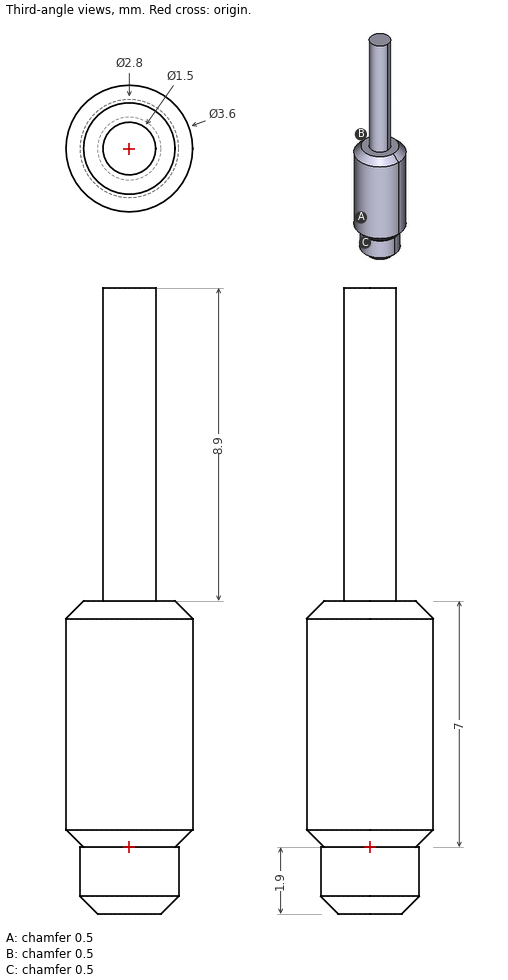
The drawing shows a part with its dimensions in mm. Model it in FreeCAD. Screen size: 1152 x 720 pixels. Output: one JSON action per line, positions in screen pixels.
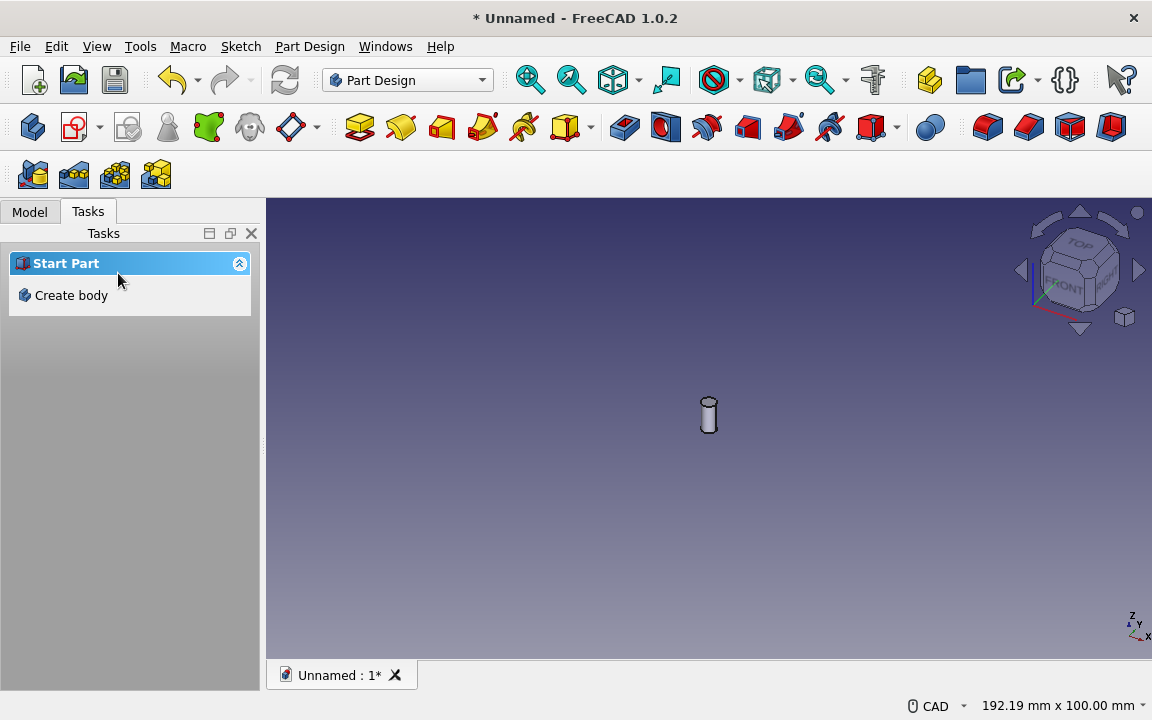
{"action": "key", "text": "v f"}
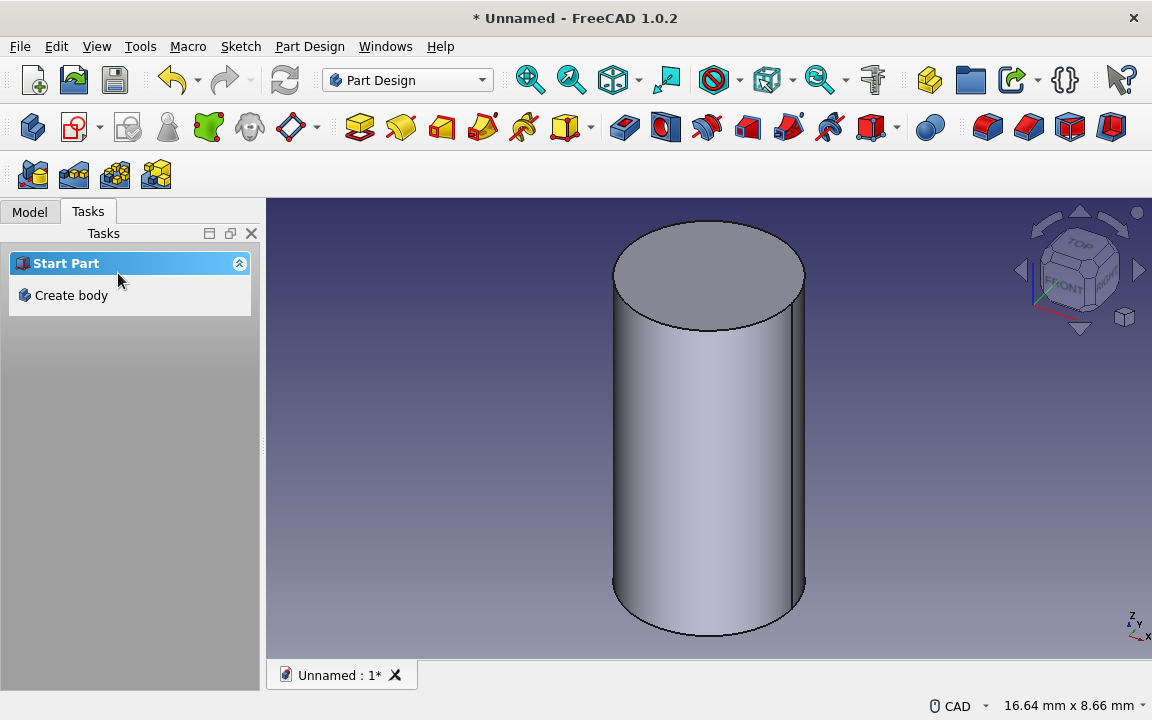
{"action": "left_click", "coordinate": [709, 275]}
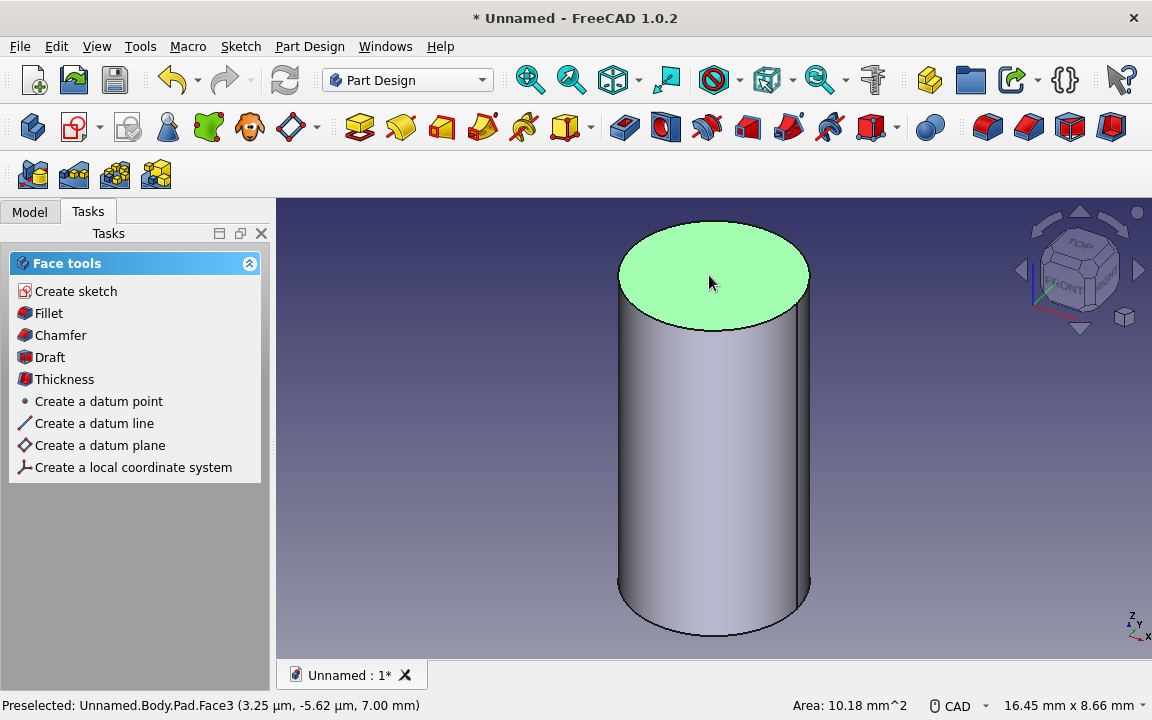
{"action": "left_click", "coordinate": [74, 128]}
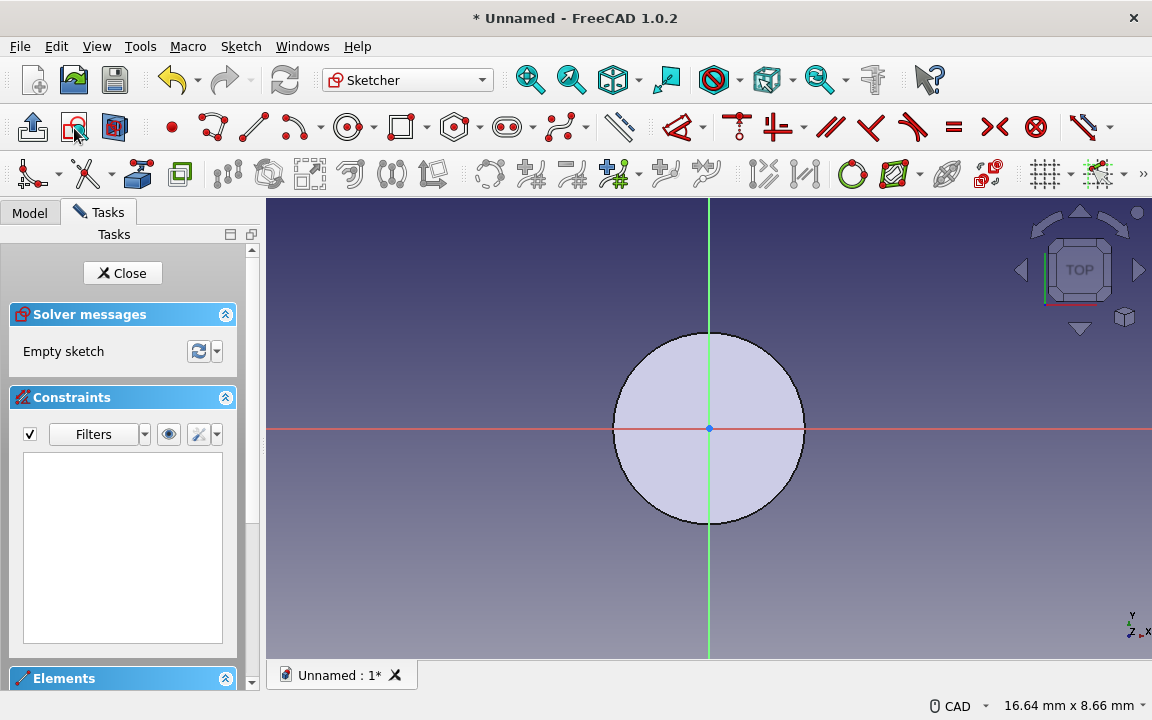
{"action": "scroll", "coordinate": [739, 428], "scroll_direction": "up", "scroll_amount": 6}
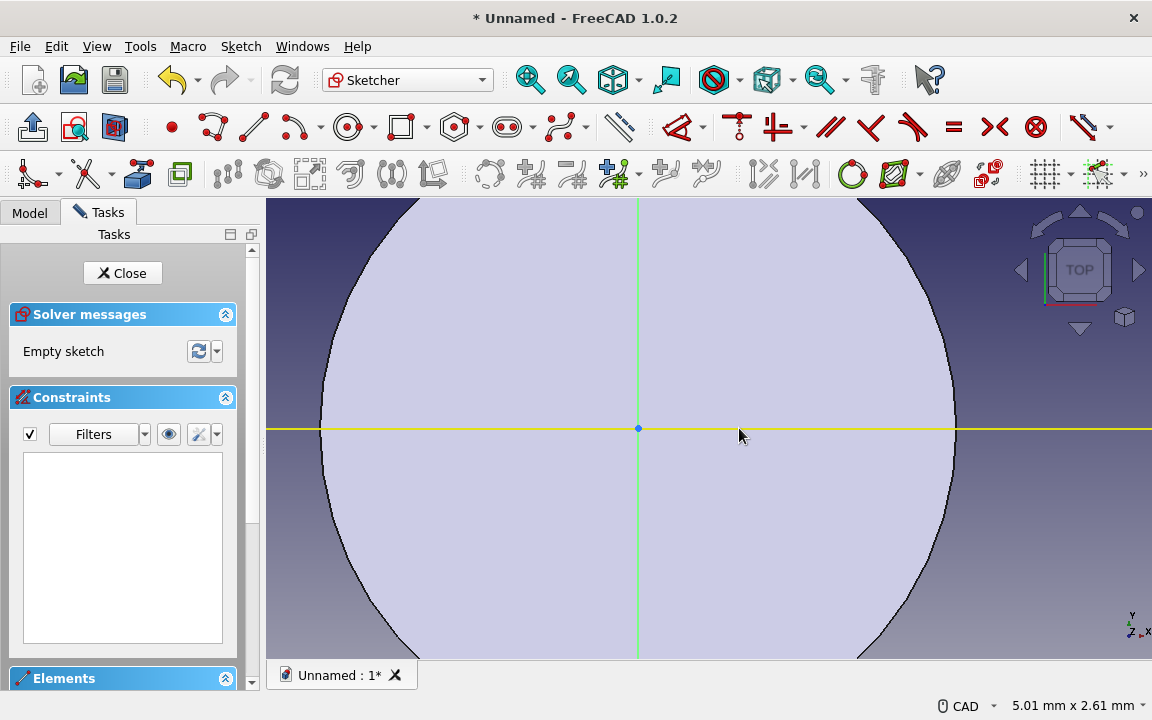
{"action": "key", "text": "g c"}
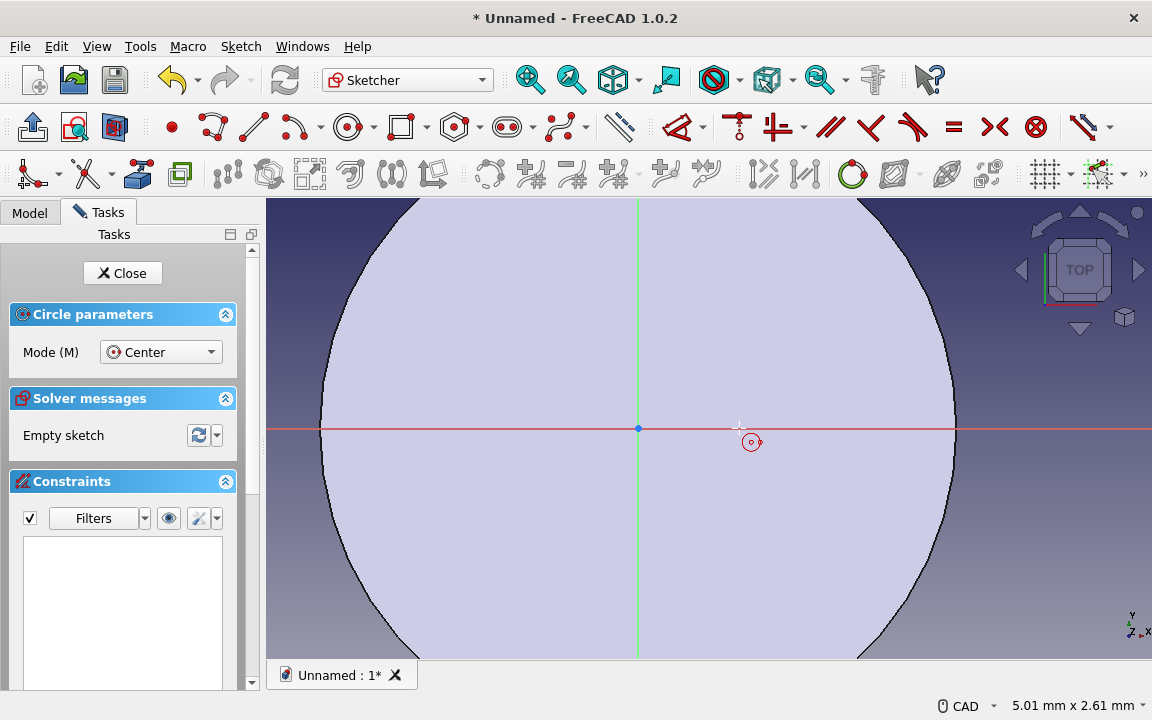
{"action": "left_click", "coordinate": [638, 428]}
{"action": "mouse_move", "coordinate": [732, 335]}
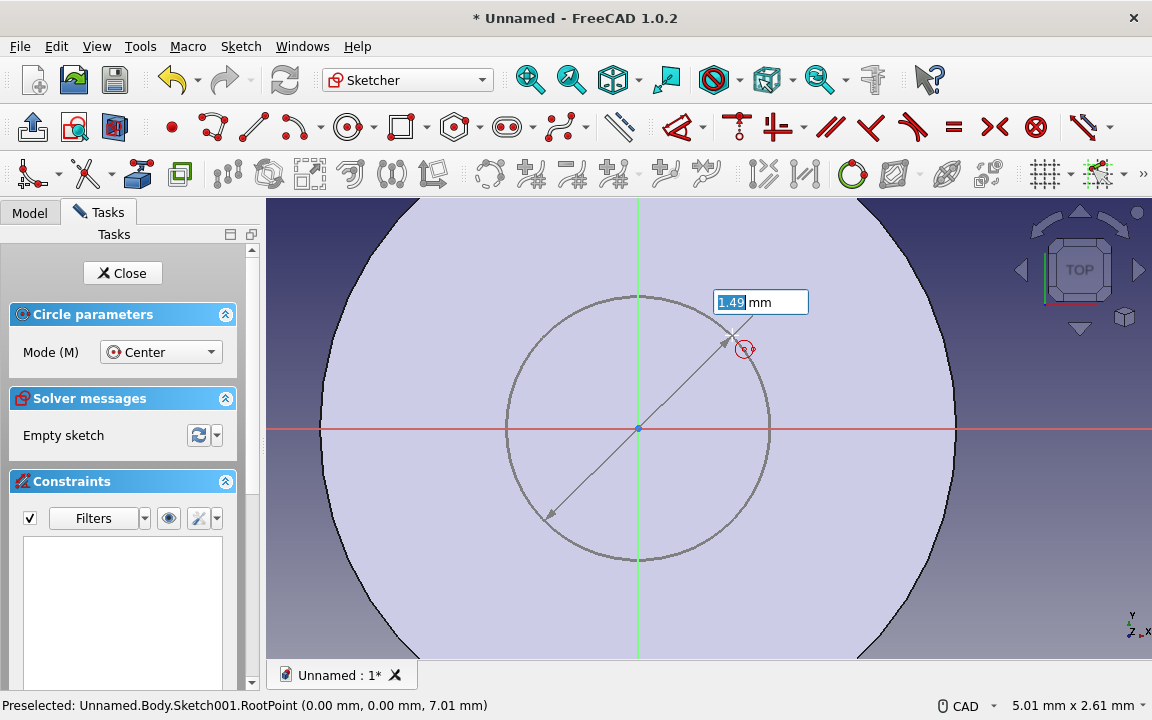
{"action": "type", "text": "1.5"}
{"action": "key", "text": "Return"}
{"action": "key", "text": "Escape"}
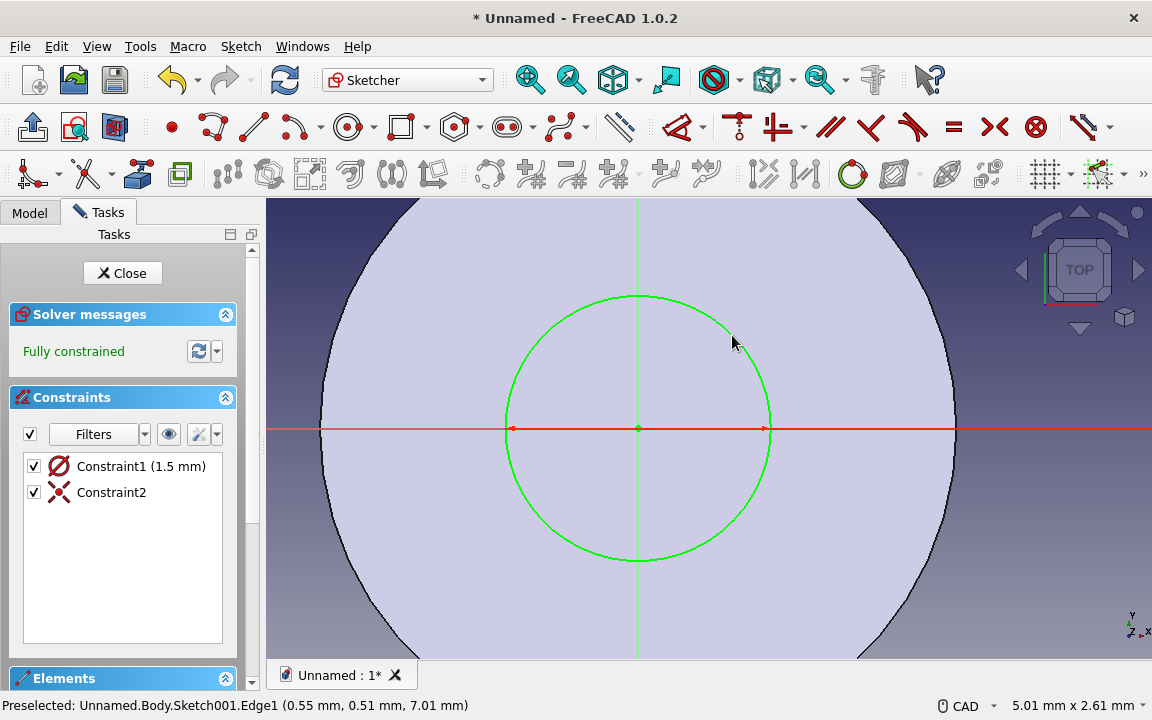
{"action": "left_click", "coordinate": [123, 273]}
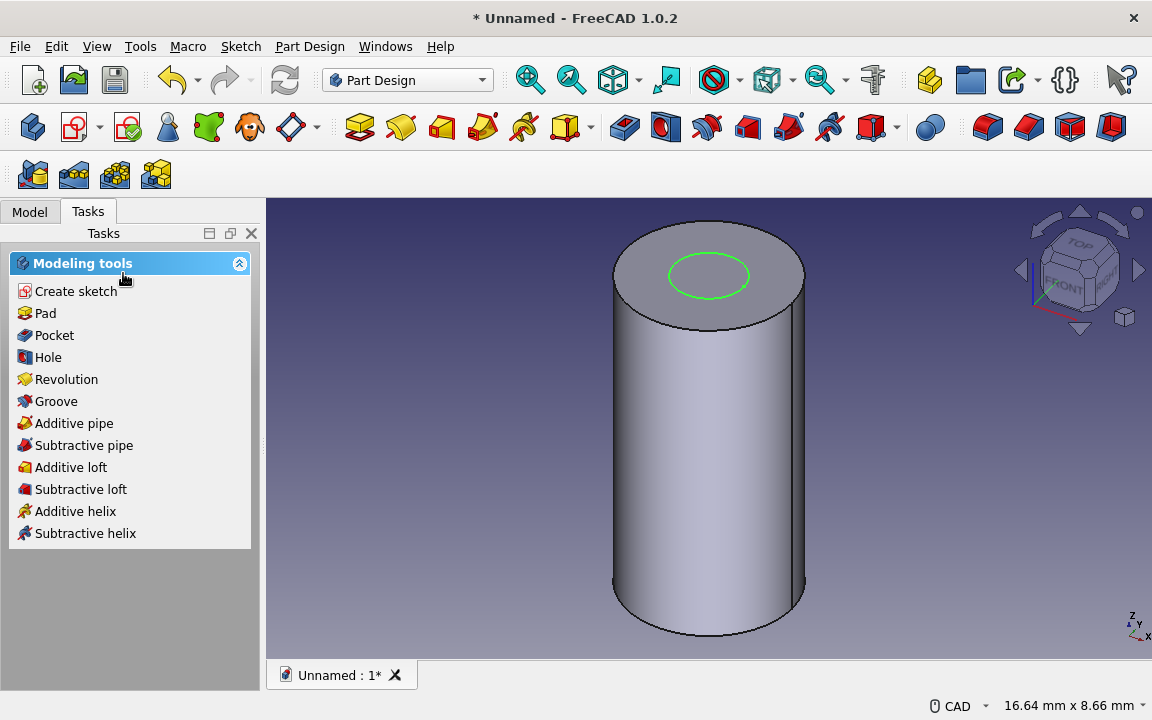
{"action": "left_click", "coordinate": [360, 128]}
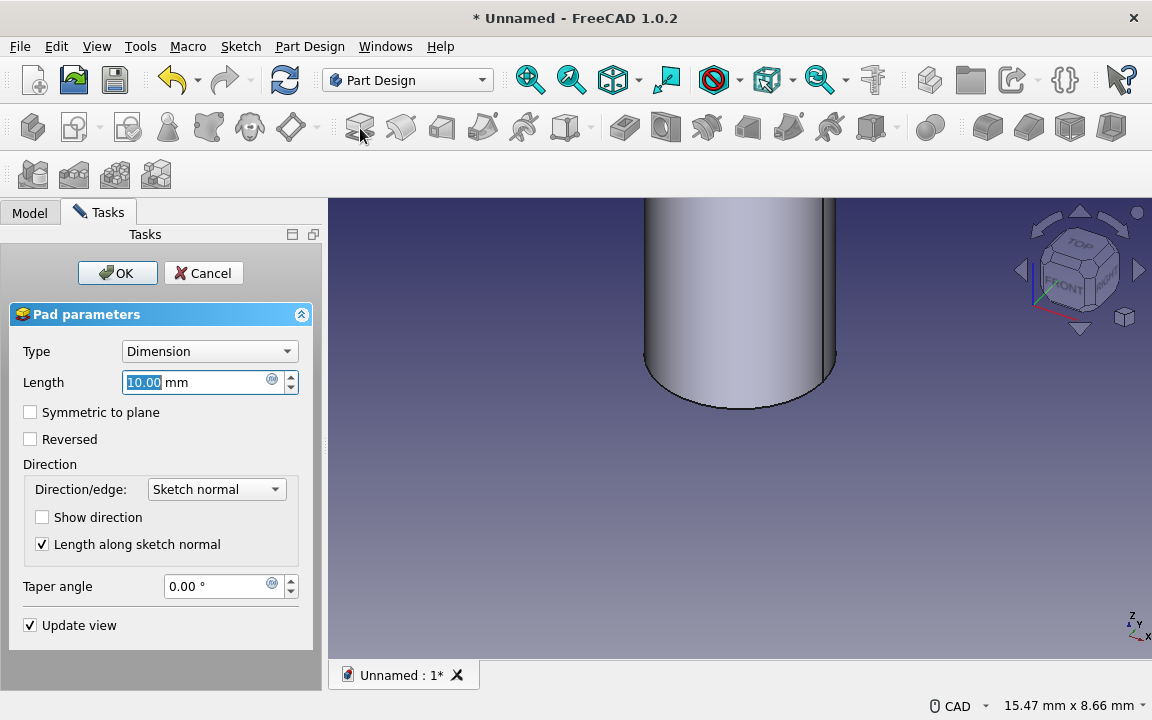
{"action": "type", "text": "8.9"}
{"action": "key", "text": "Tab"}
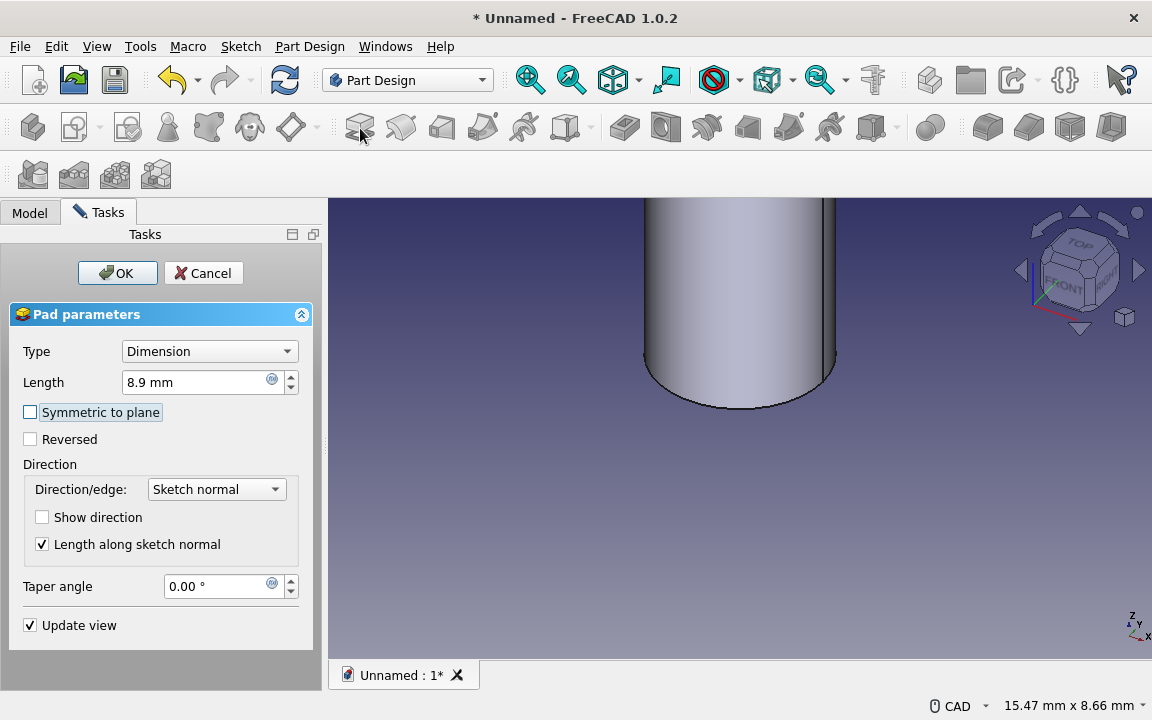
{"action": "left_click", "coordinate": [118, 273]}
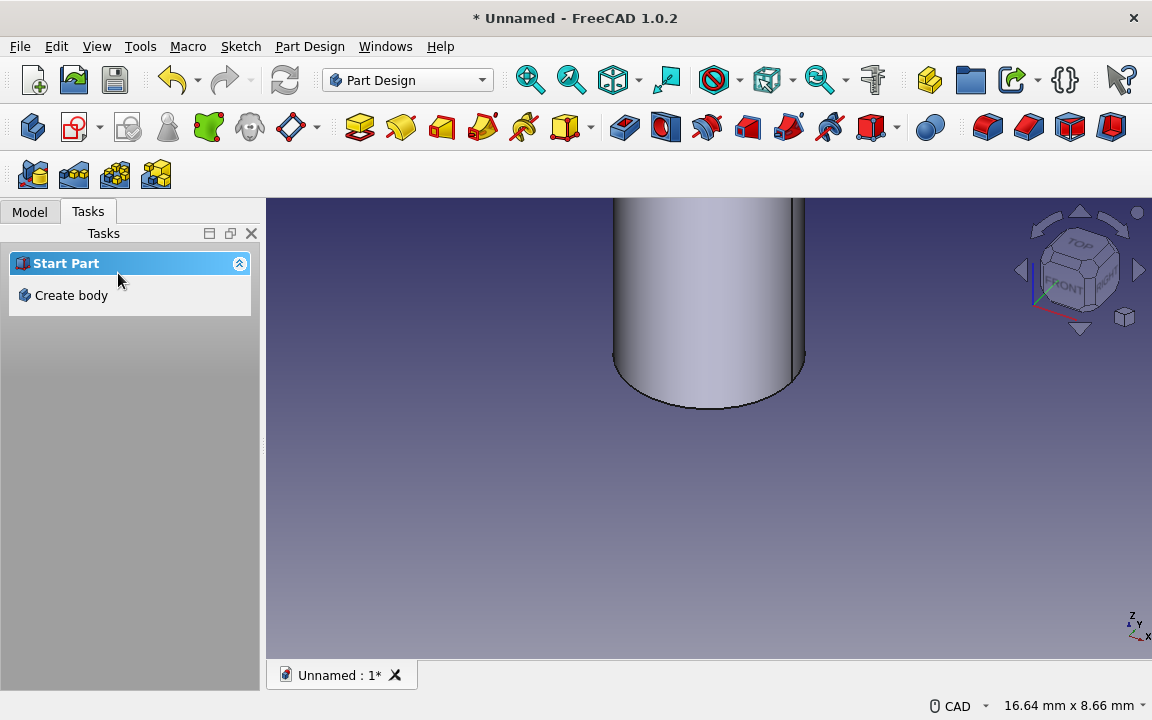
{"action": "key", "text": "v f"}